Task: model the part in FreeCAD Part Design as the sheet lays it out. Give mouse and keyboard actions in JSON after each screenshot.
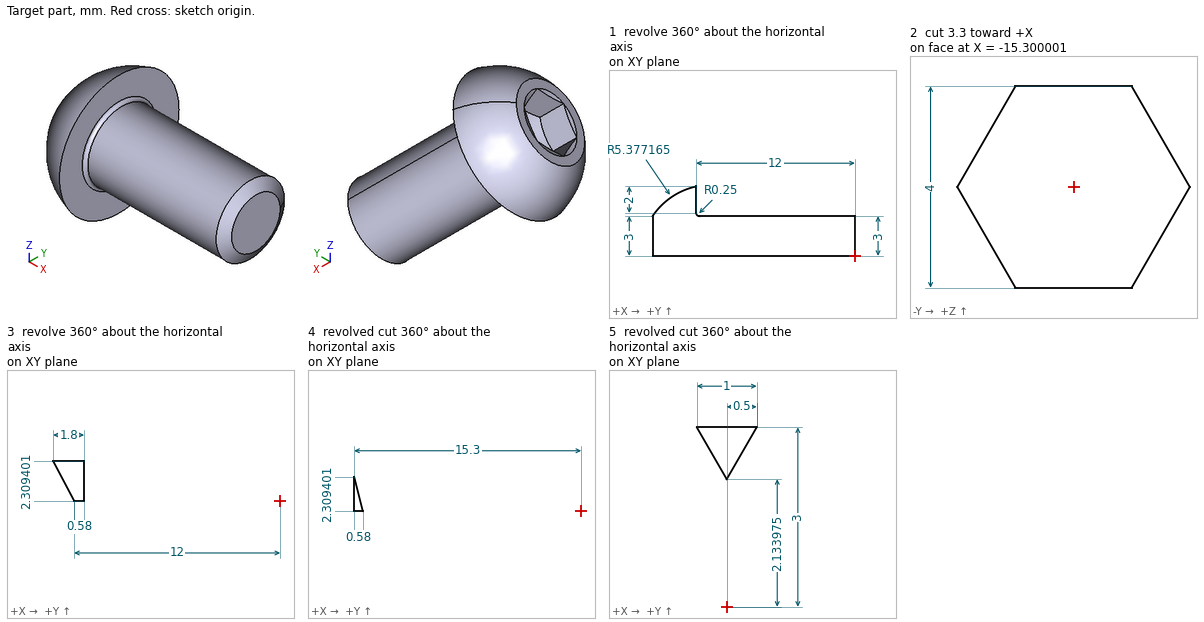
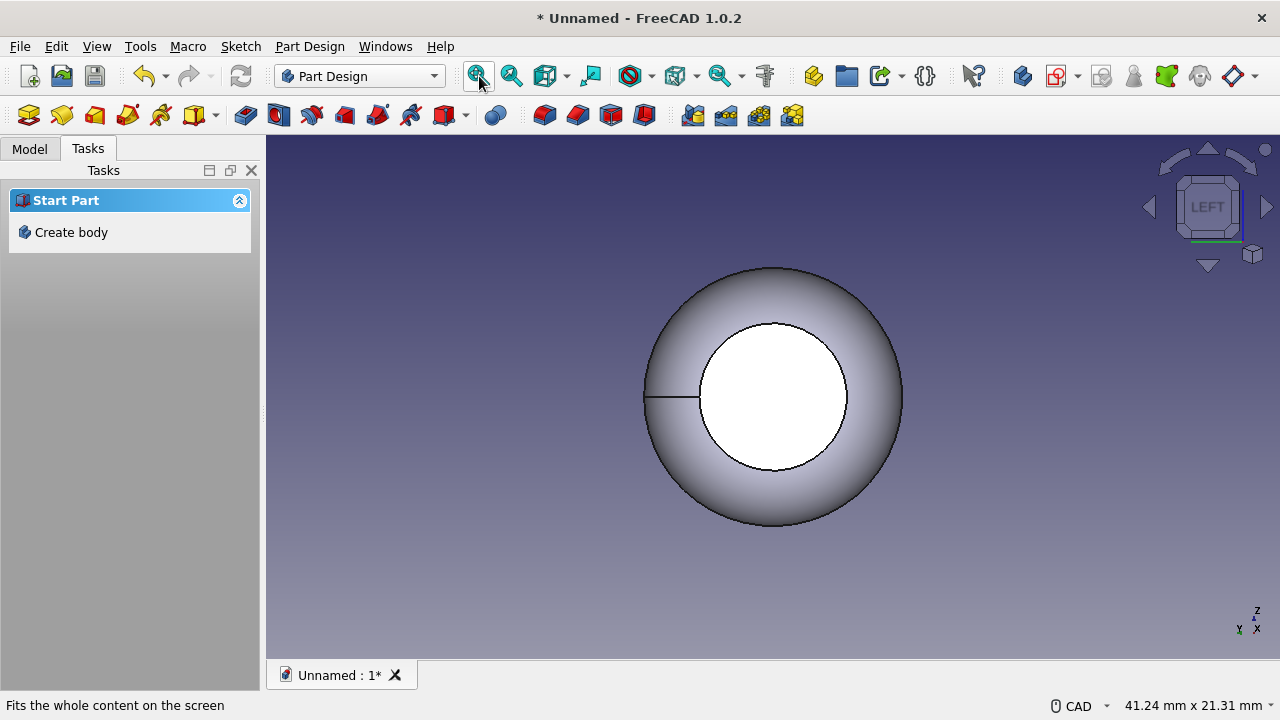
{"action": "left_click", "coordinate": [773, 396]}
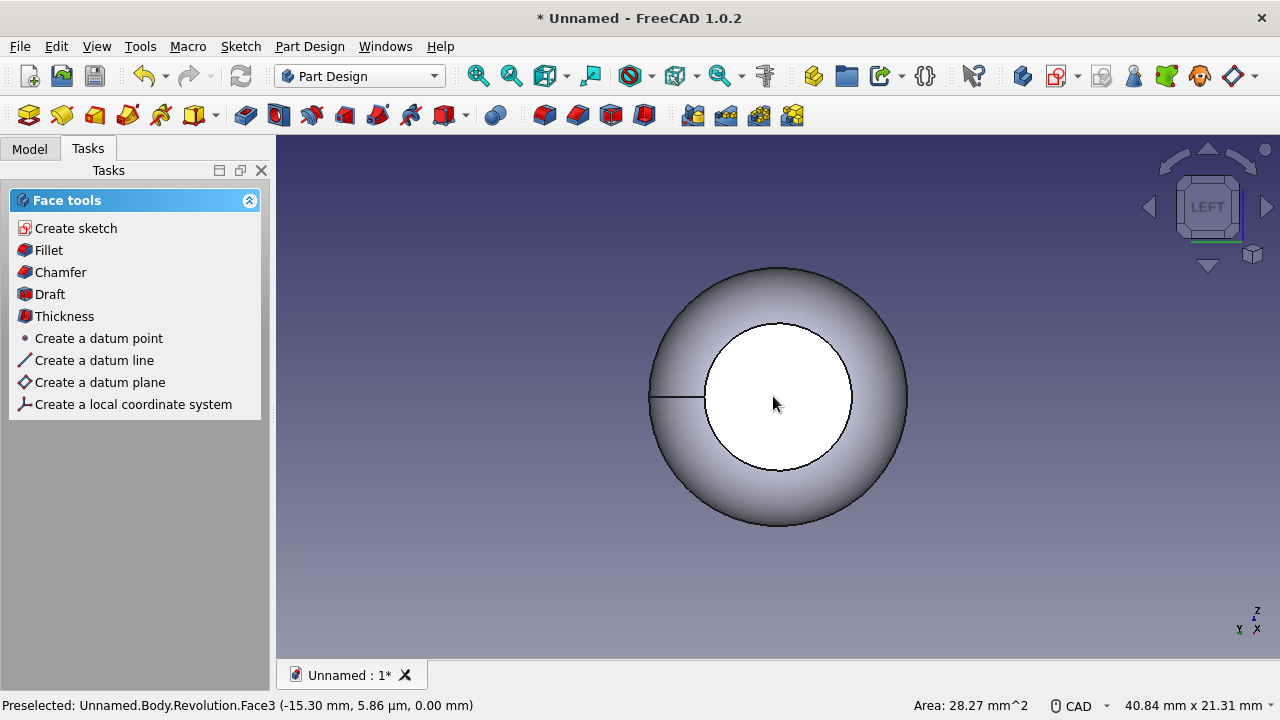
{"action": "left_click", "coordinate": [1056, 76]}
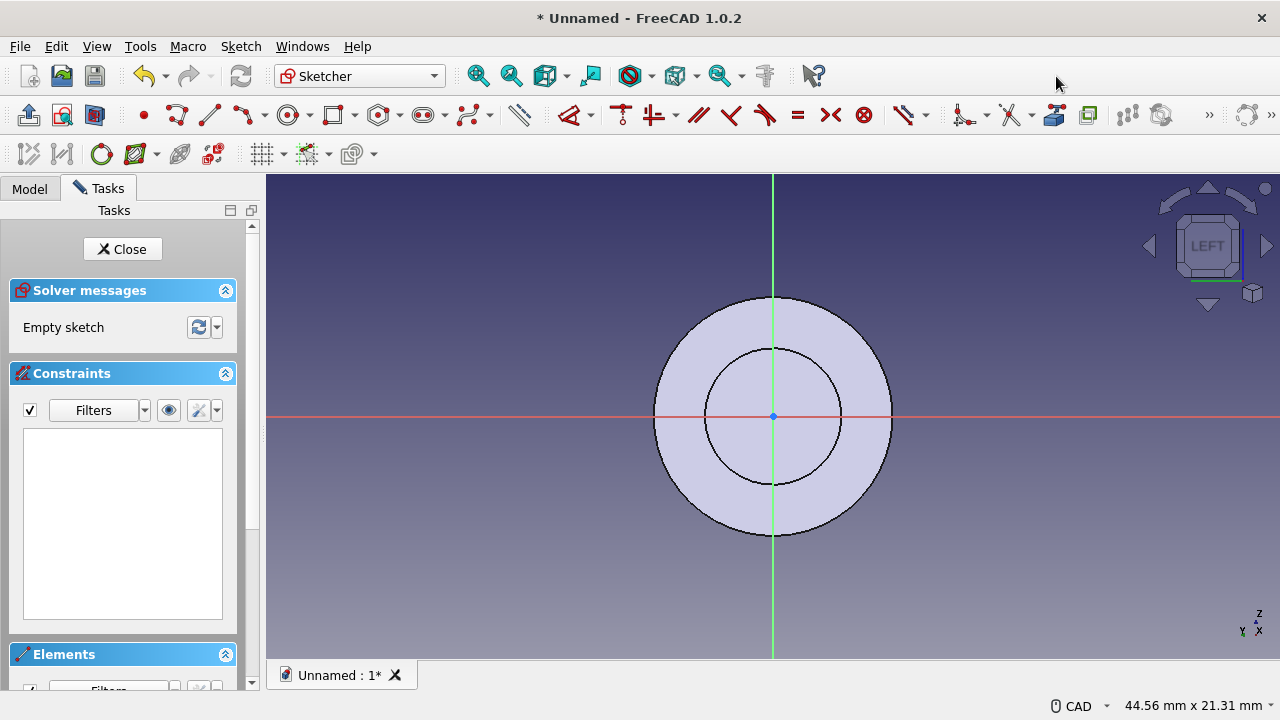
{"action": "scroll", "coordinate": [803, 416], "scroll_direction": "up", "scroll_amount": 6}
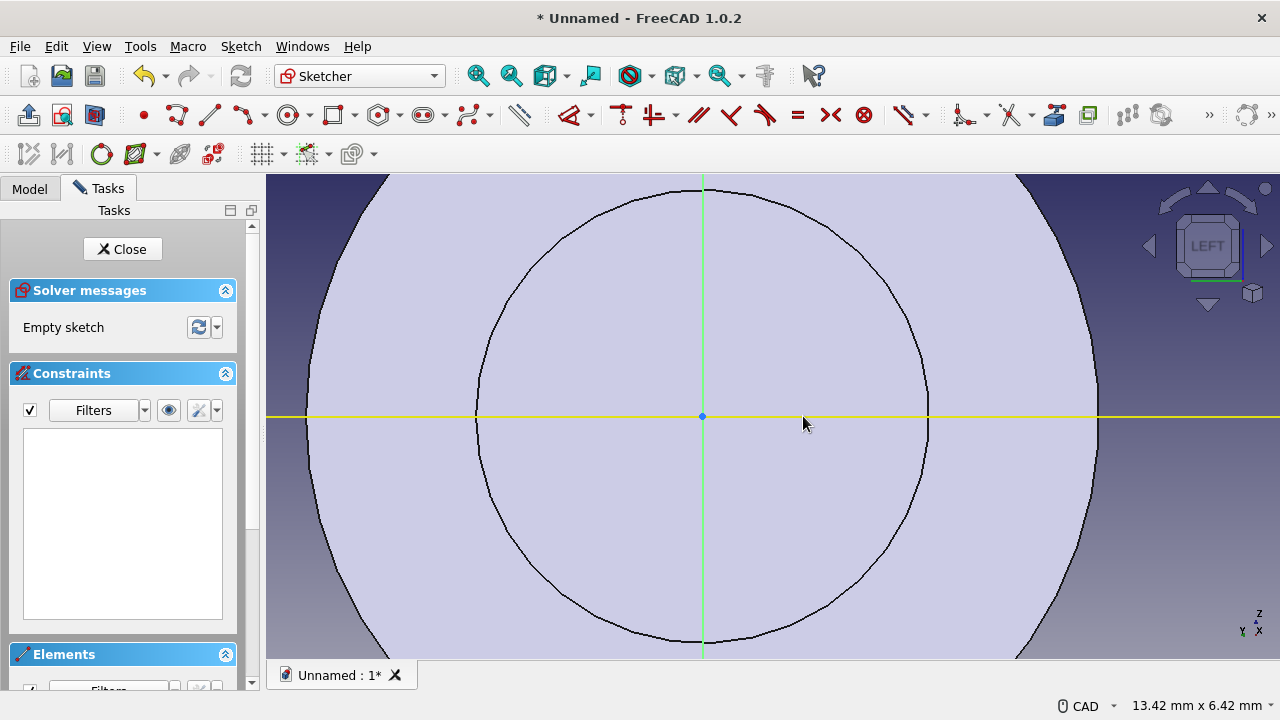
{"action": "left_click", "coordinate": [378, 116]}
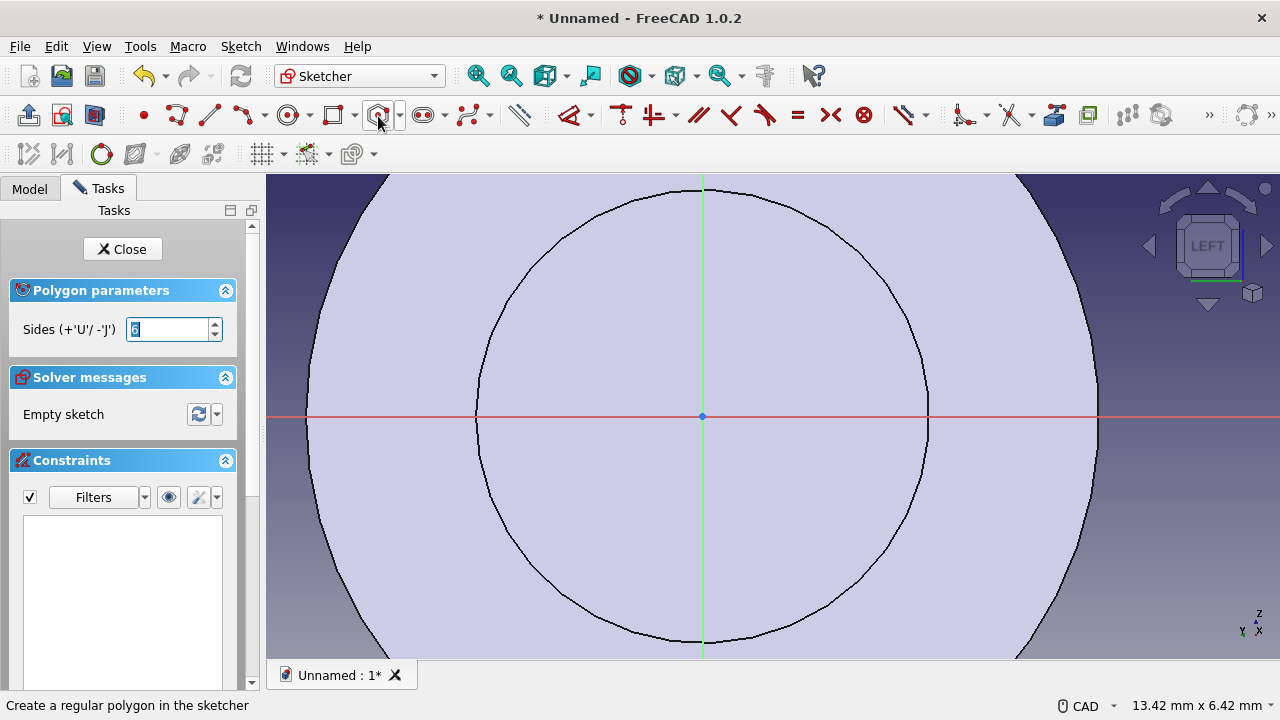
{"action": "left_click", "coordinate": [703, 416]}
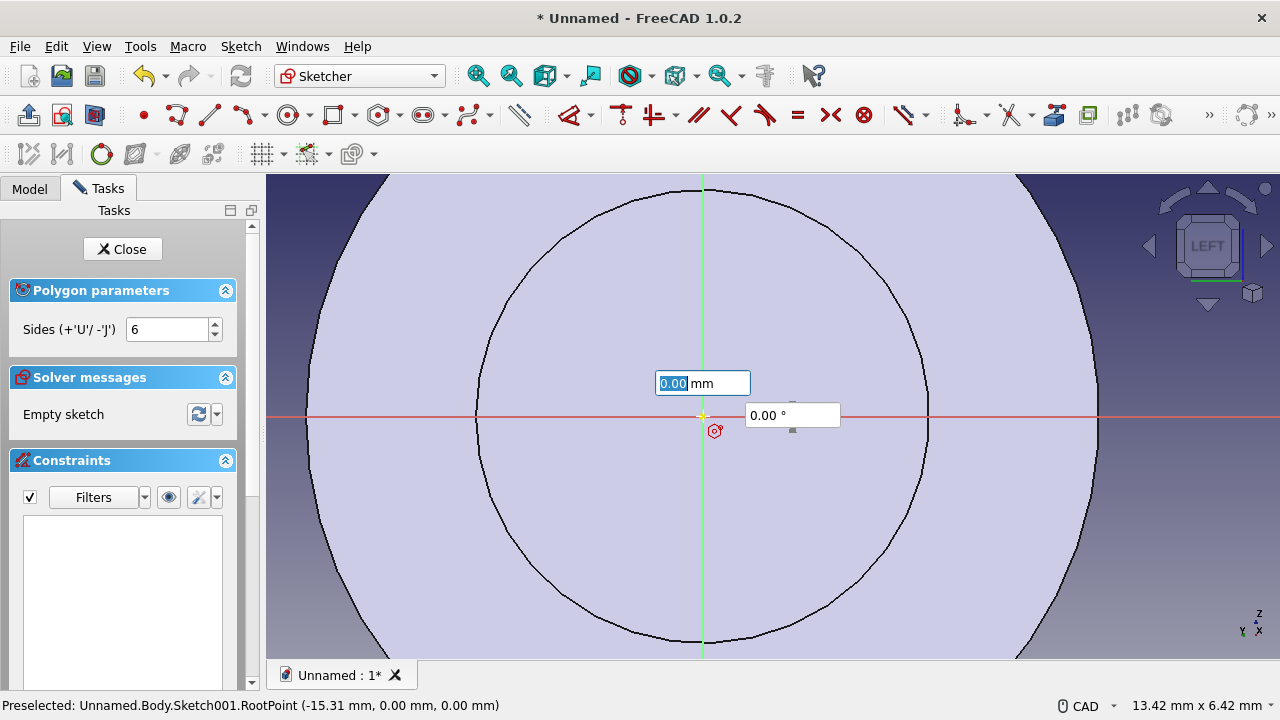
{"action": "left_click", "coordinate": [528, 416]}
{"action": "key", "text": "Escape"}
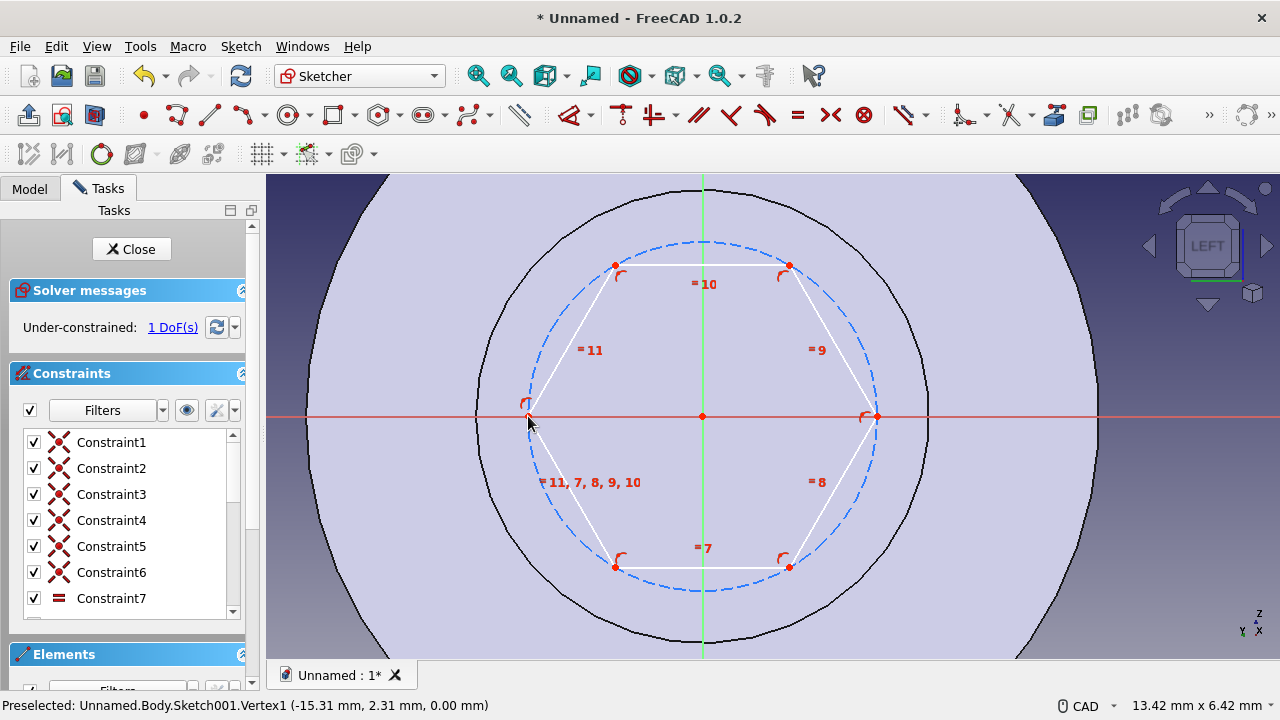
{"action": "left_click", "coordinate": [568, 116]}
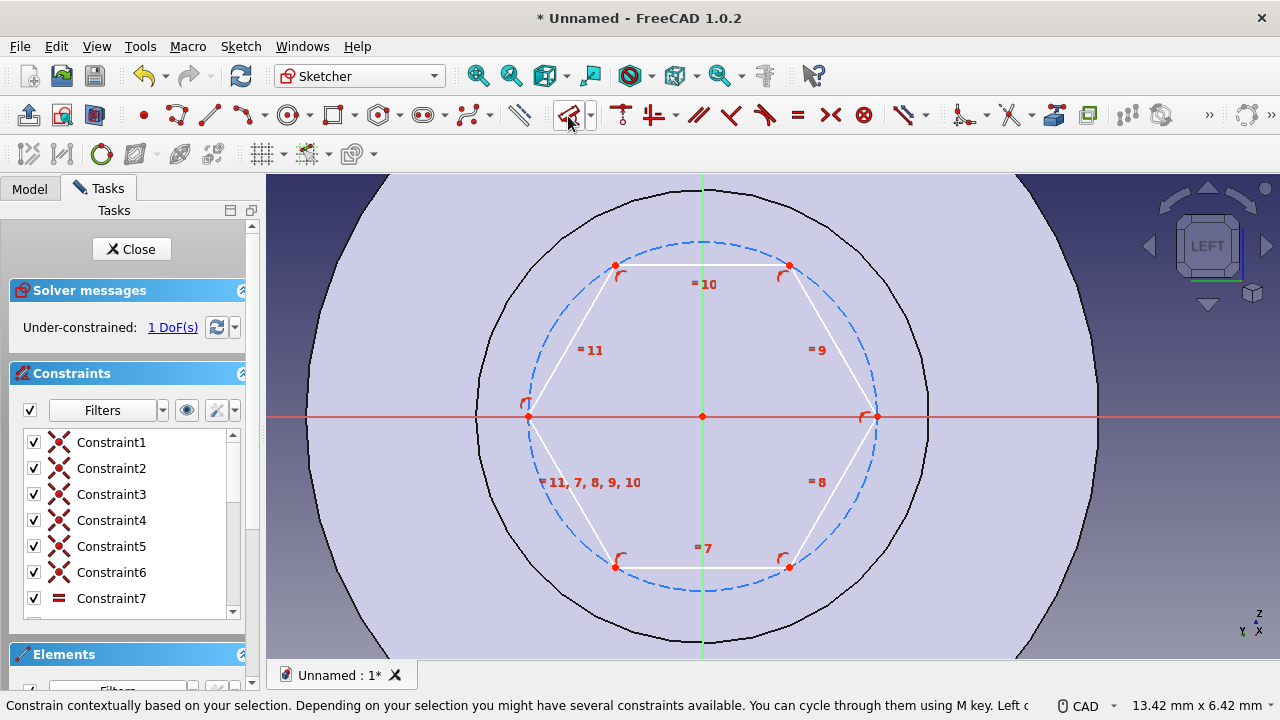
{"action": "left_click", "coordinate": [615, 568]}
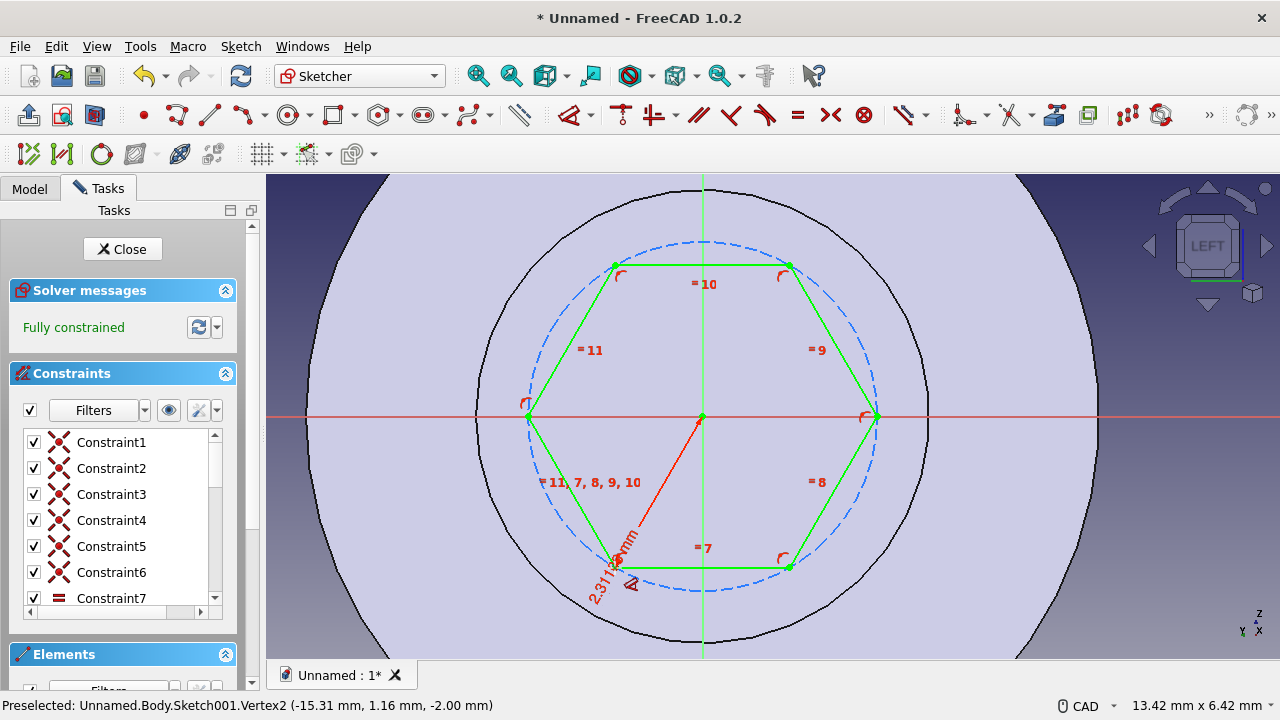
{"action": "left_click", "coordinate": [790, 265]}
{"action": "left_click", "coordinate": [872, 311]}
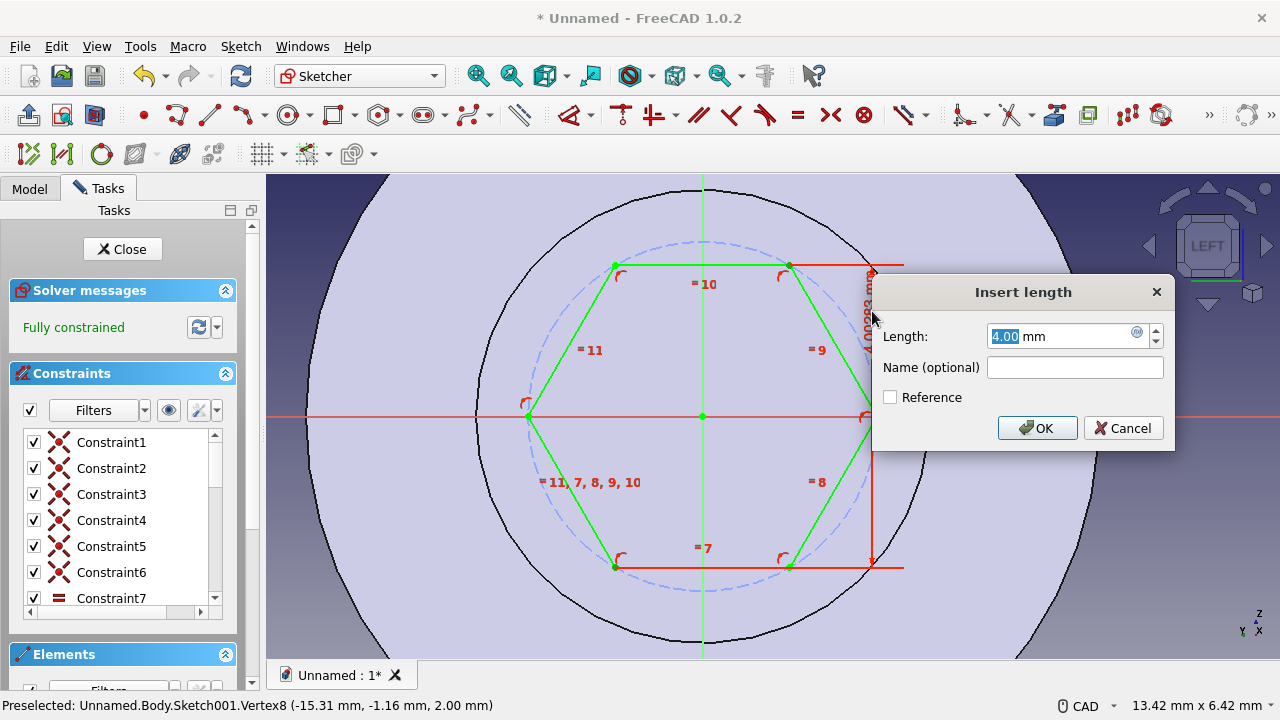
{"action": "type", "text": "4"}
{"action": "key", "text": "Return"}
{"action": "key", "text": "Escape"}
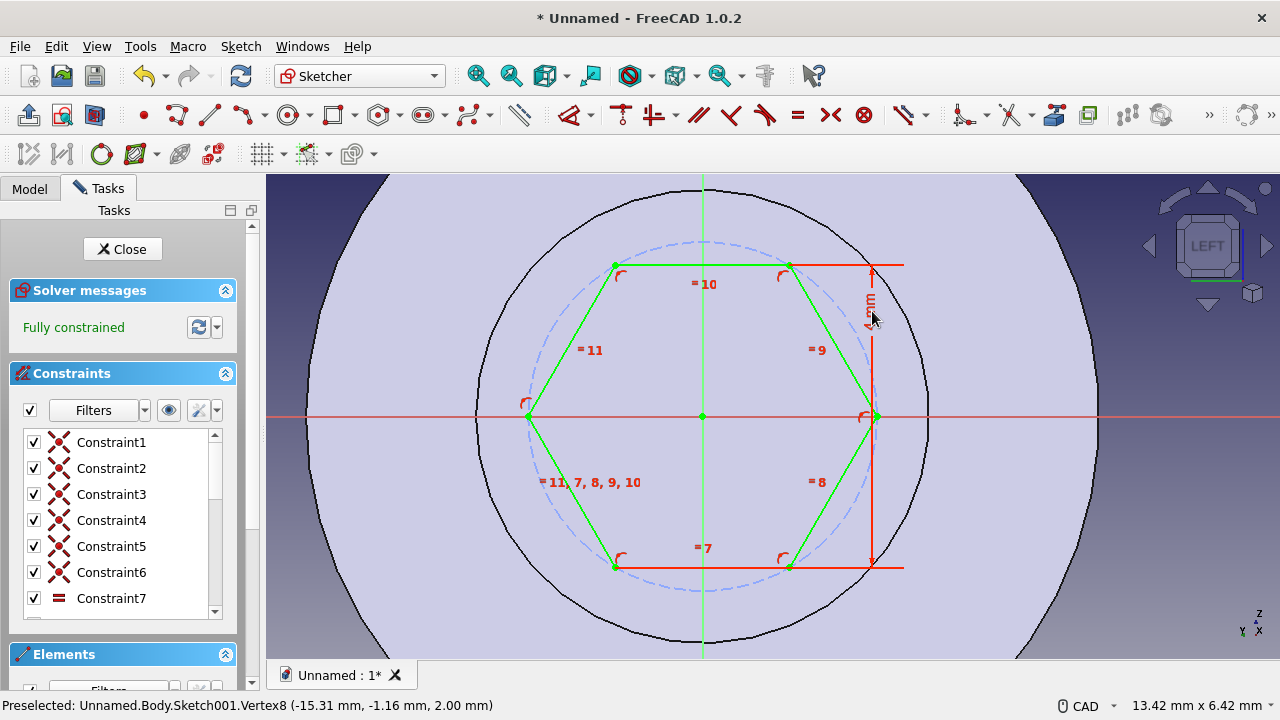
{"action": "left_click", "coordinate": [123, 249]}